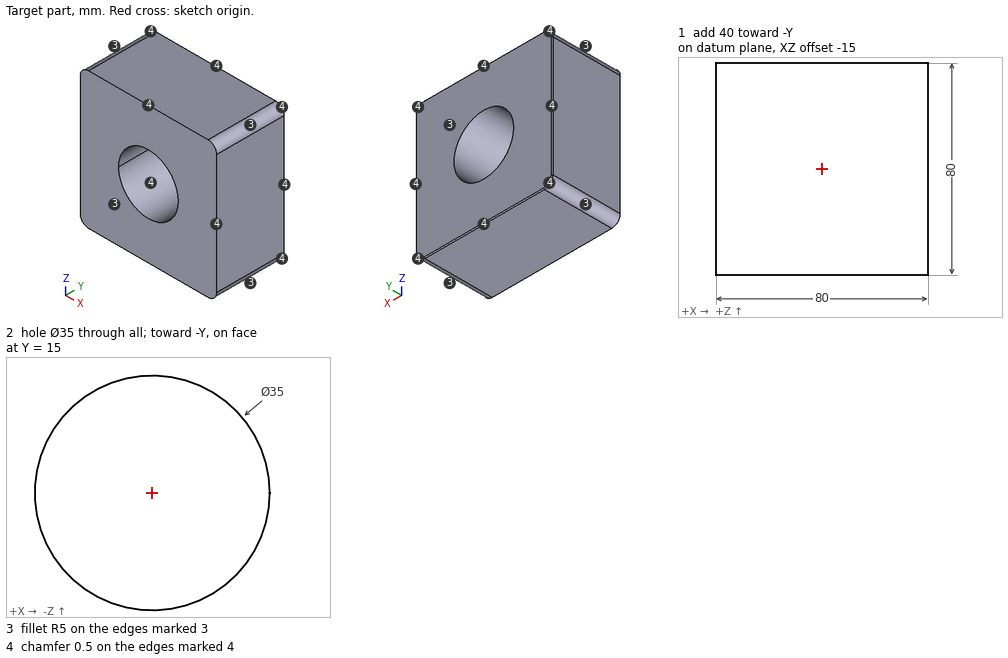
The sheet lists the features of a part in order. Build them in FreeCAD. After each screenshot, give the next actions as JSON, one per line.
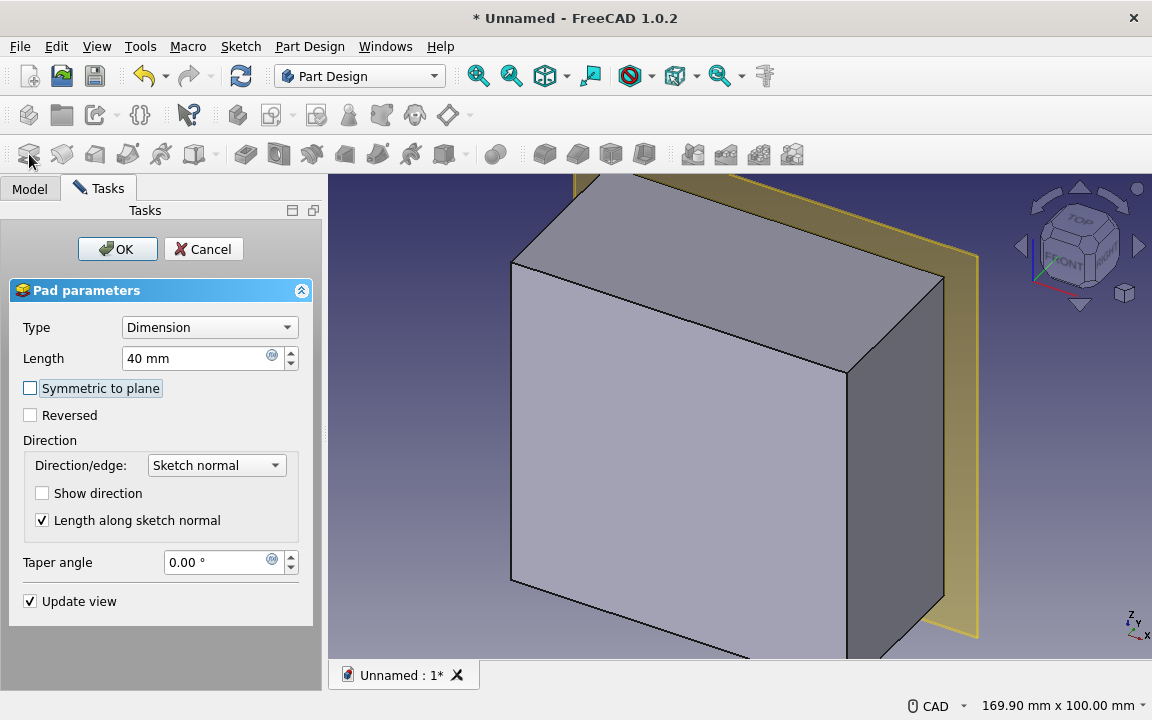
{"action": "left_click", "coordinate": [118, 249]}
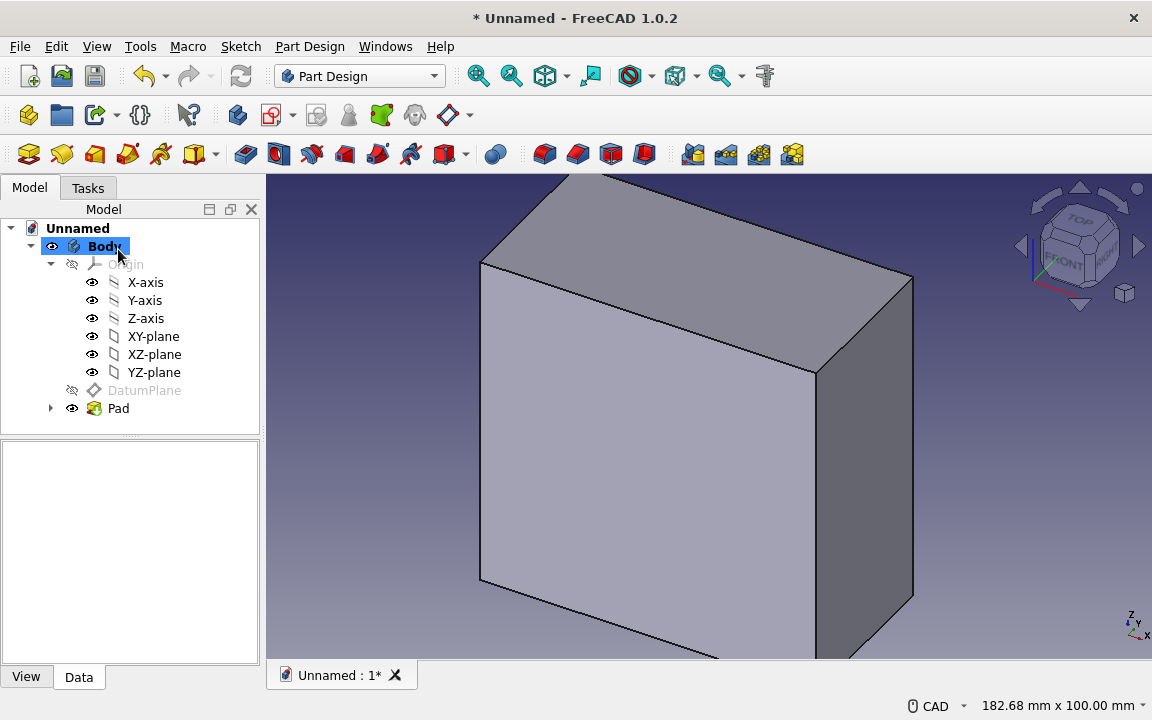
{"action": "left_click", "coordinate": [479, 76]}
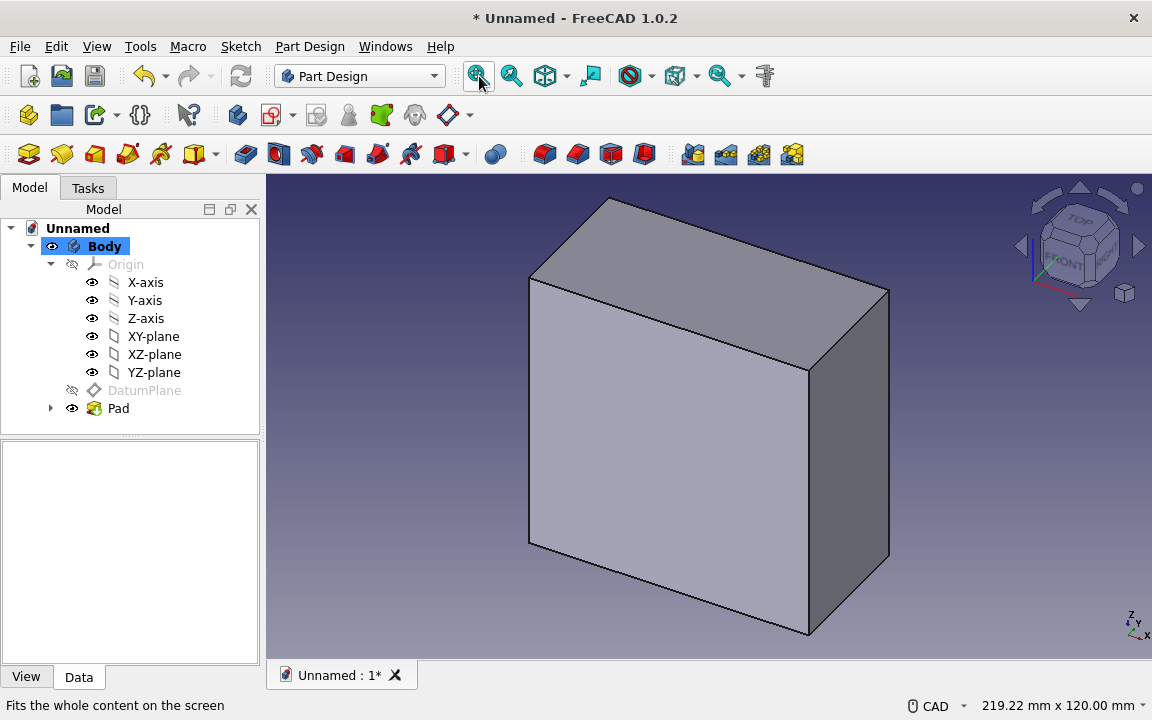
{"action": "key", "text": "4"}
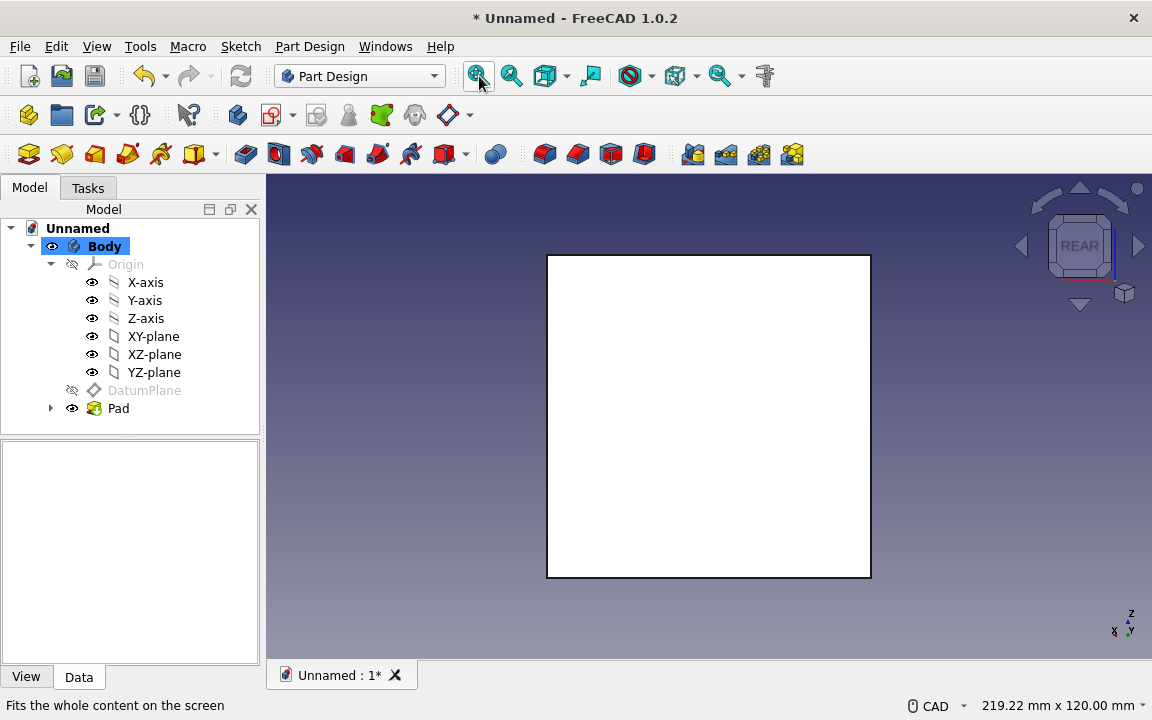
{"action": "left_click", "coordinate": [709, 416]}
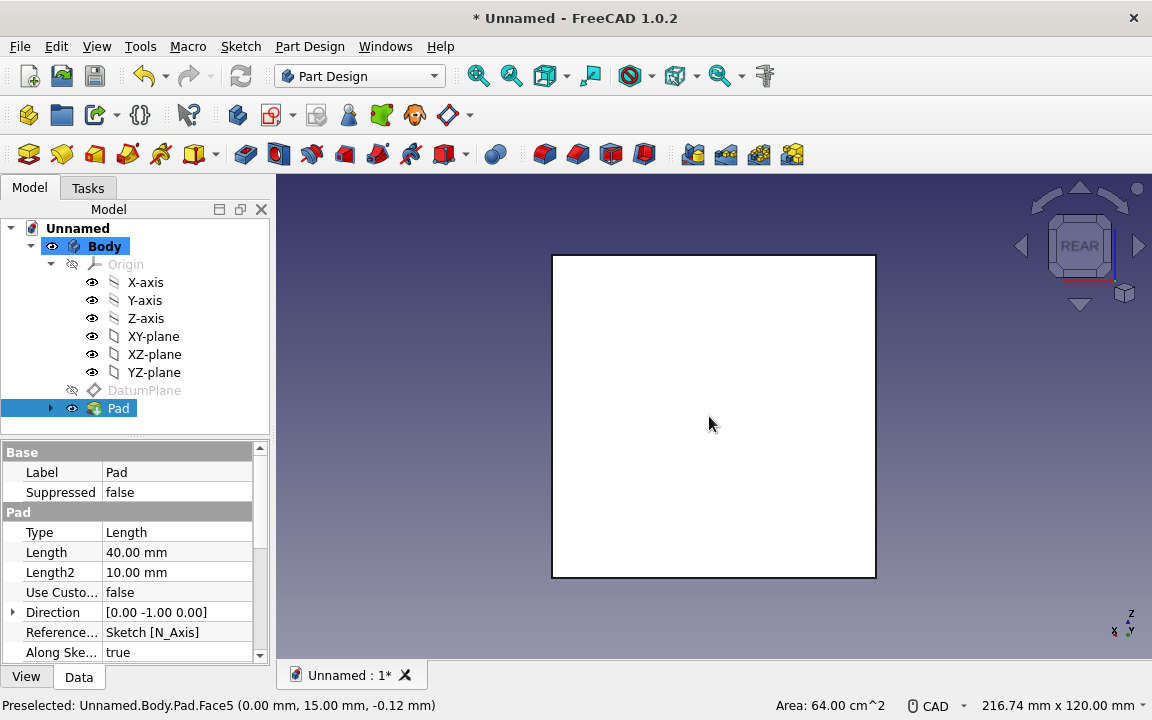
{"action": "left_click", "coordinate": [270, 116]}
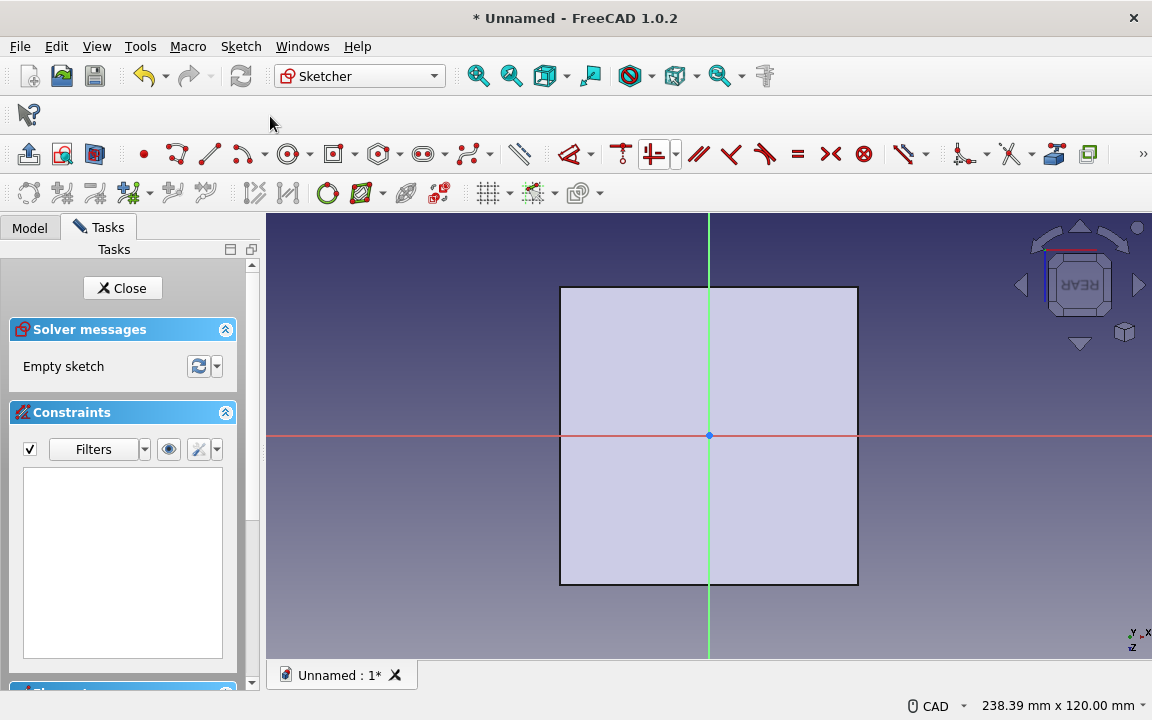
{"action": "scroll", "coordinate": [765, 436], "scroll_direction": "up", "scroll_amount": 4}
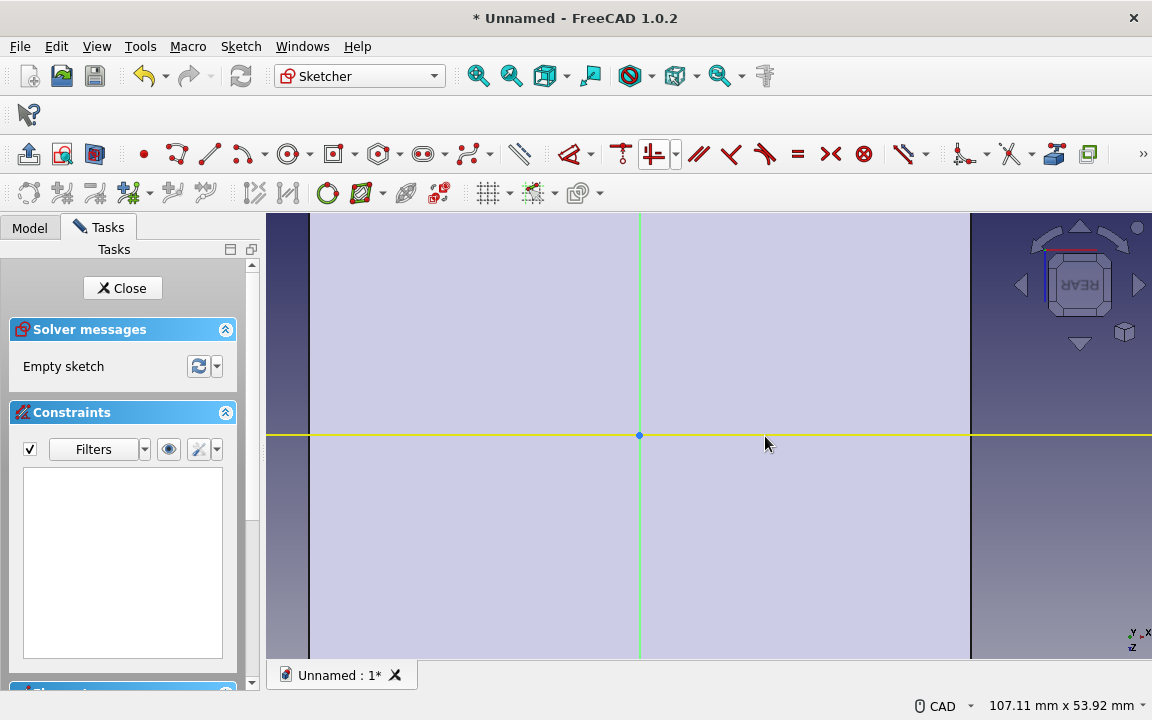
{"action": "left_click", "coordinate": [288, 154]}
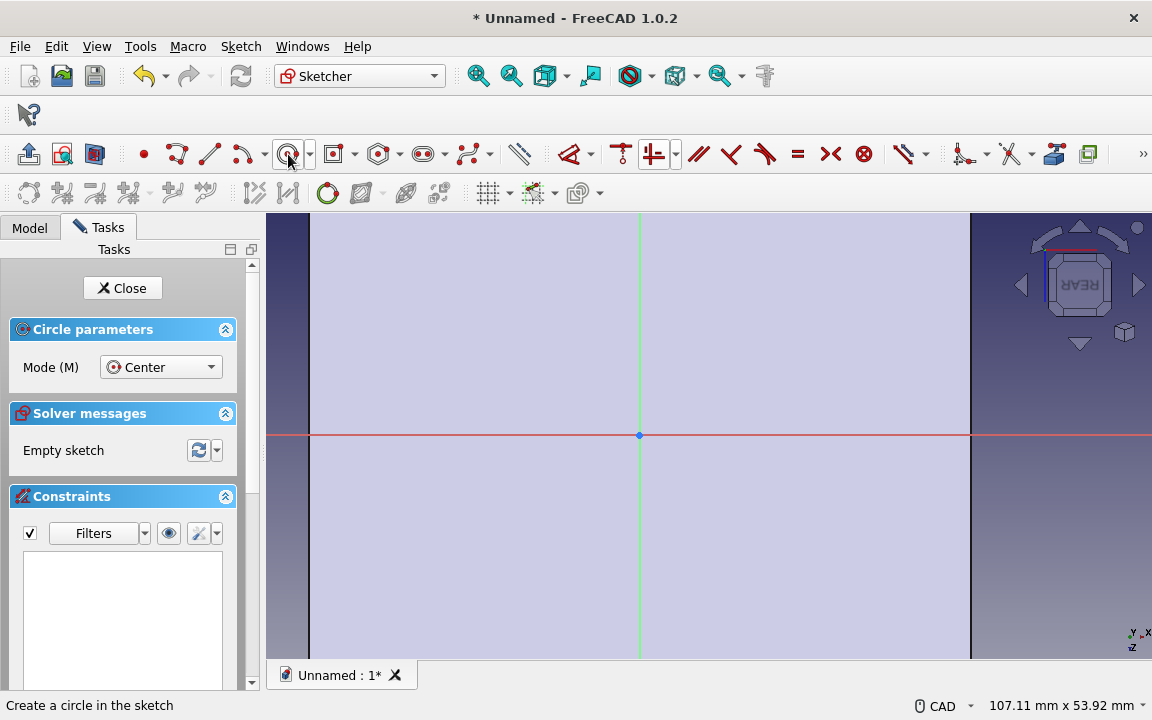
{"action": "left_click", "coordinate": [640, 435]}
{"action": "left_click", "coordinate": [742, 333]}
{"action": "key", "text": "Escape"}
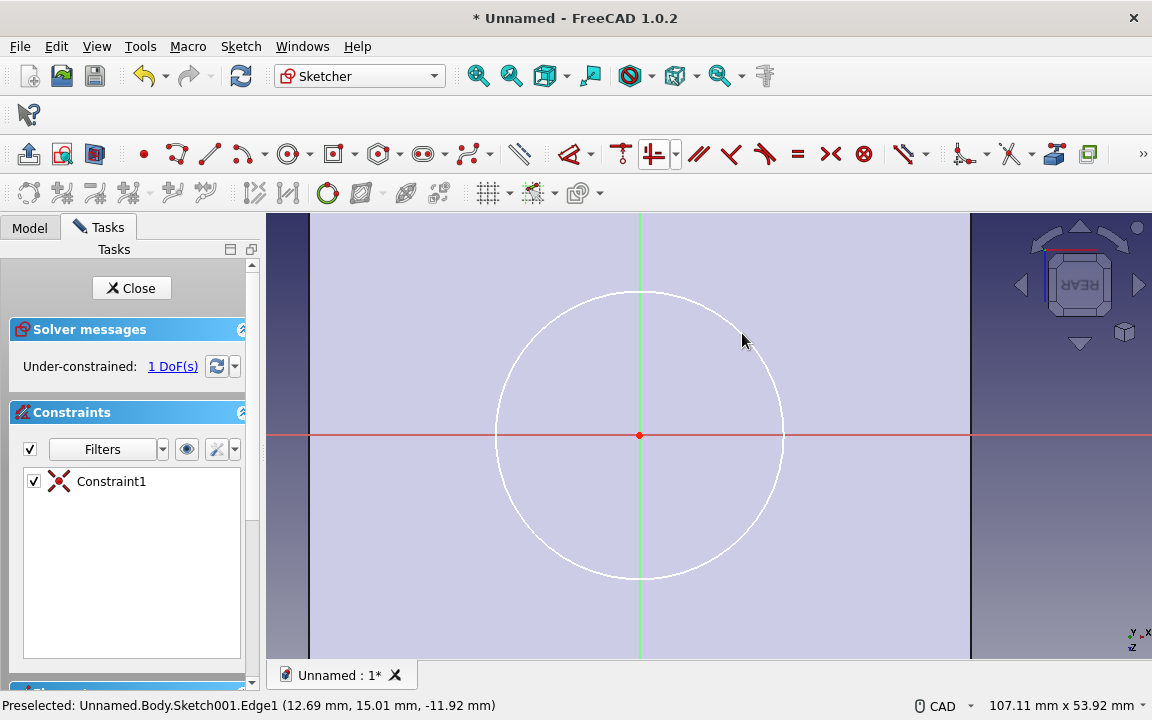
{"action": "key", "text": "d"}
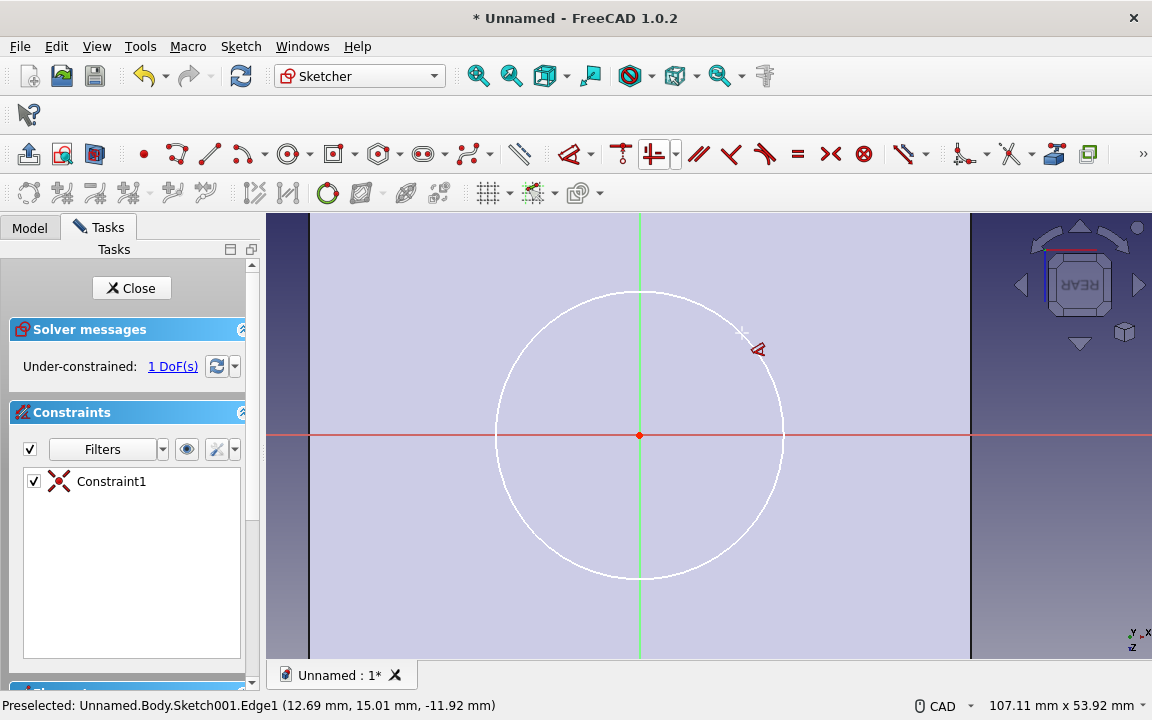
{"action": "left_click", "coordinate": [741, 333]}
{"action": "left_click", "coordinate": [764, 310]}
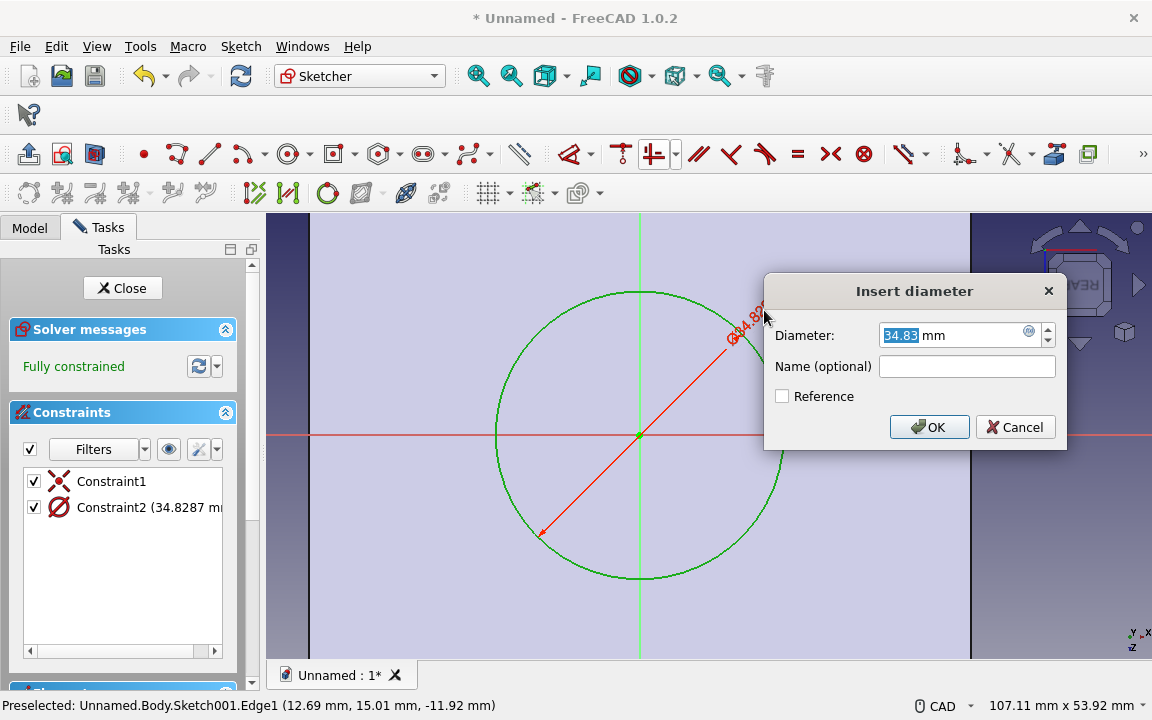
{"action": "type", "text": "35"}
{"action": "key", "text": "Return"}
{"action": "key", "text": "Escape"}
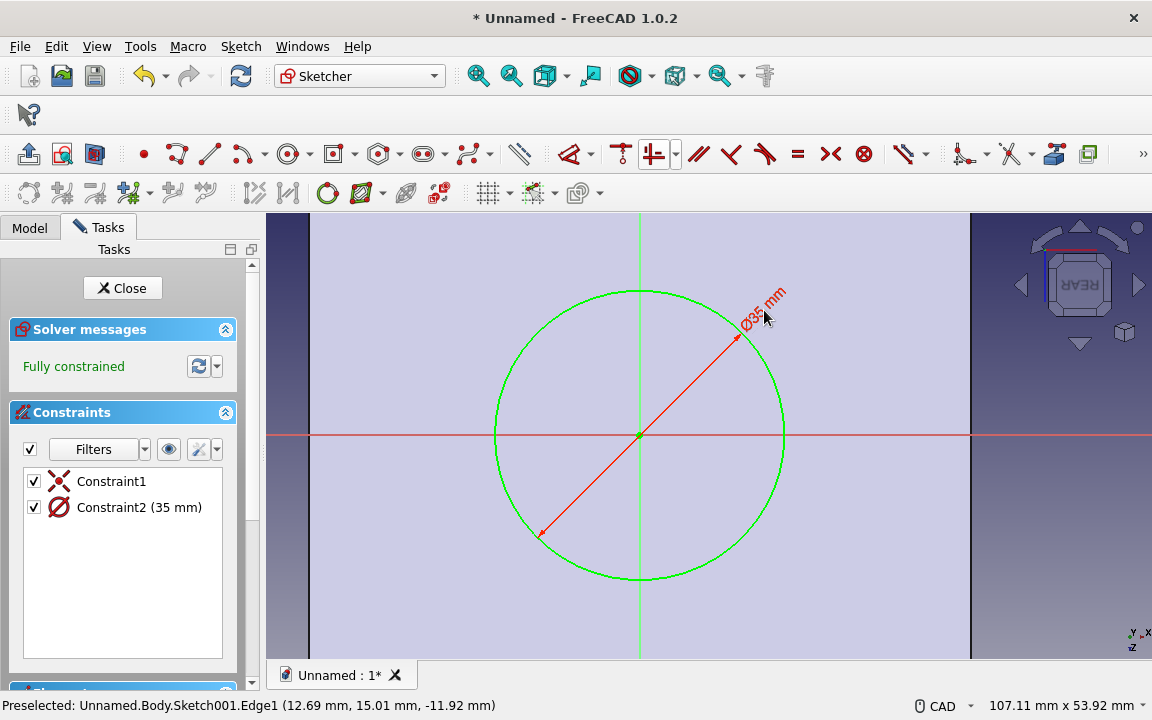
{"action": "left_click", "coordinate": [123, 288]}